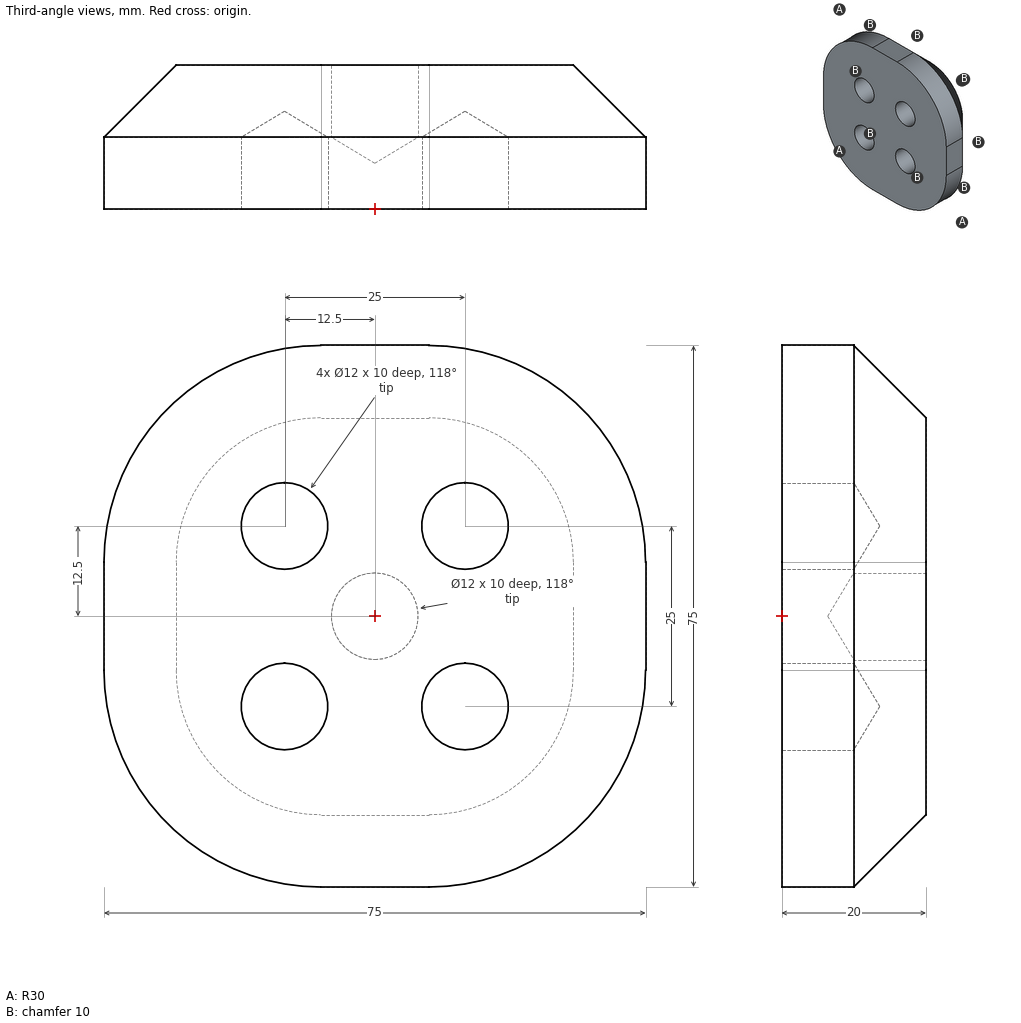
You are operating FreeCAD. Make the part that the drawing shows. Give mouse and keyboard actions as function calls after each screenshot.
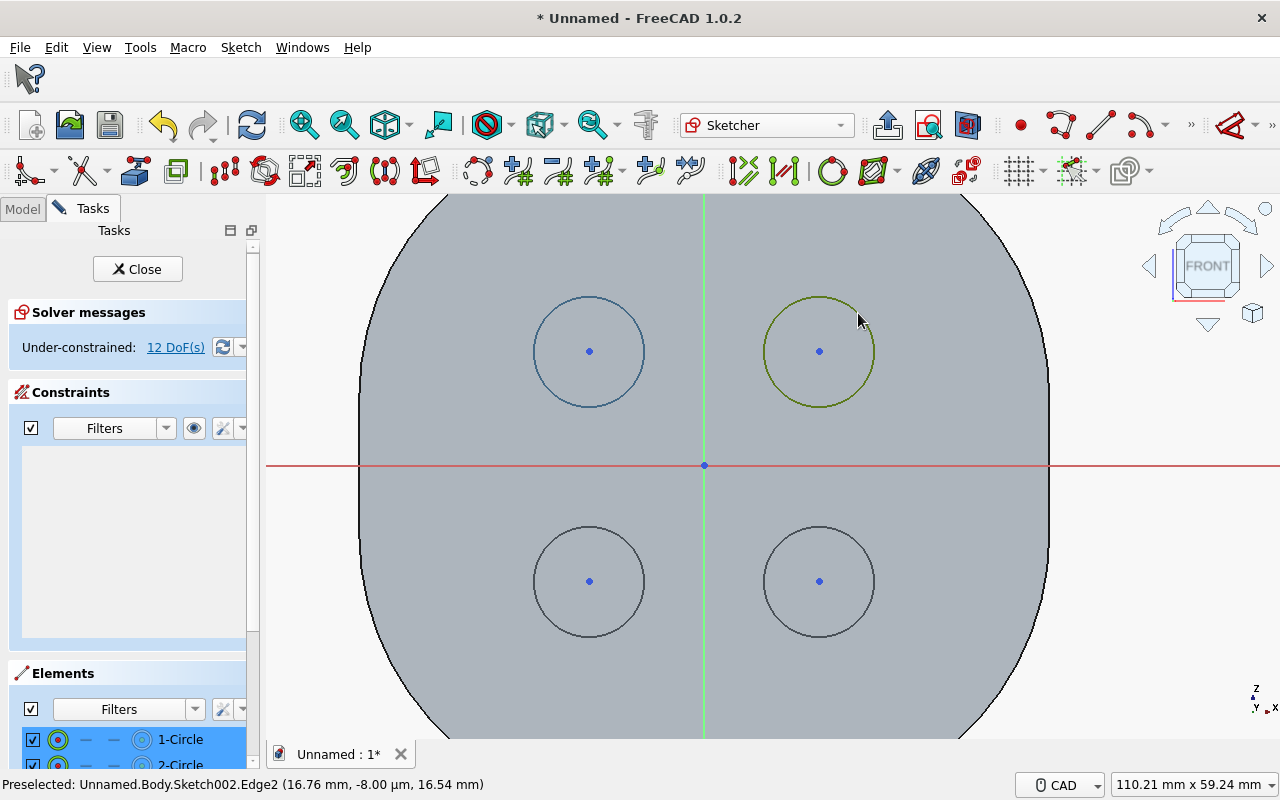
click(858, 543)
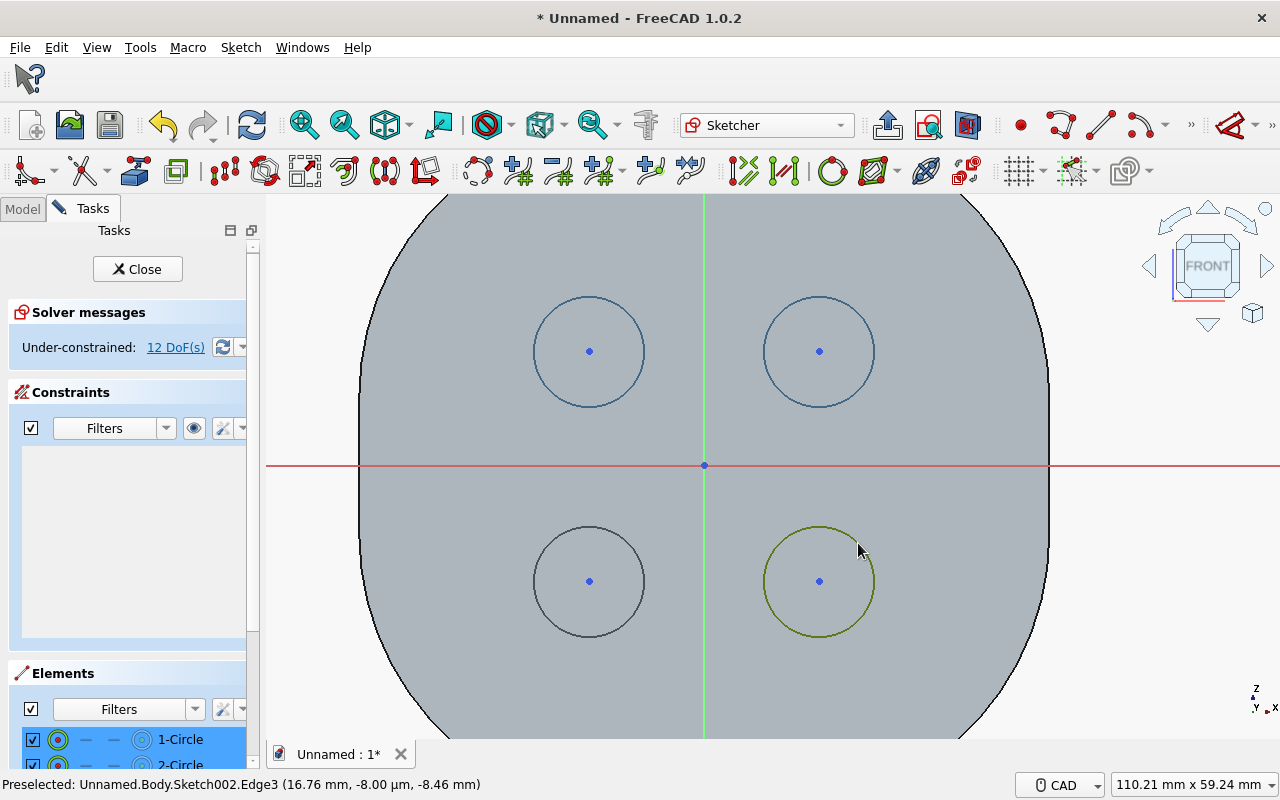
click(628, 543)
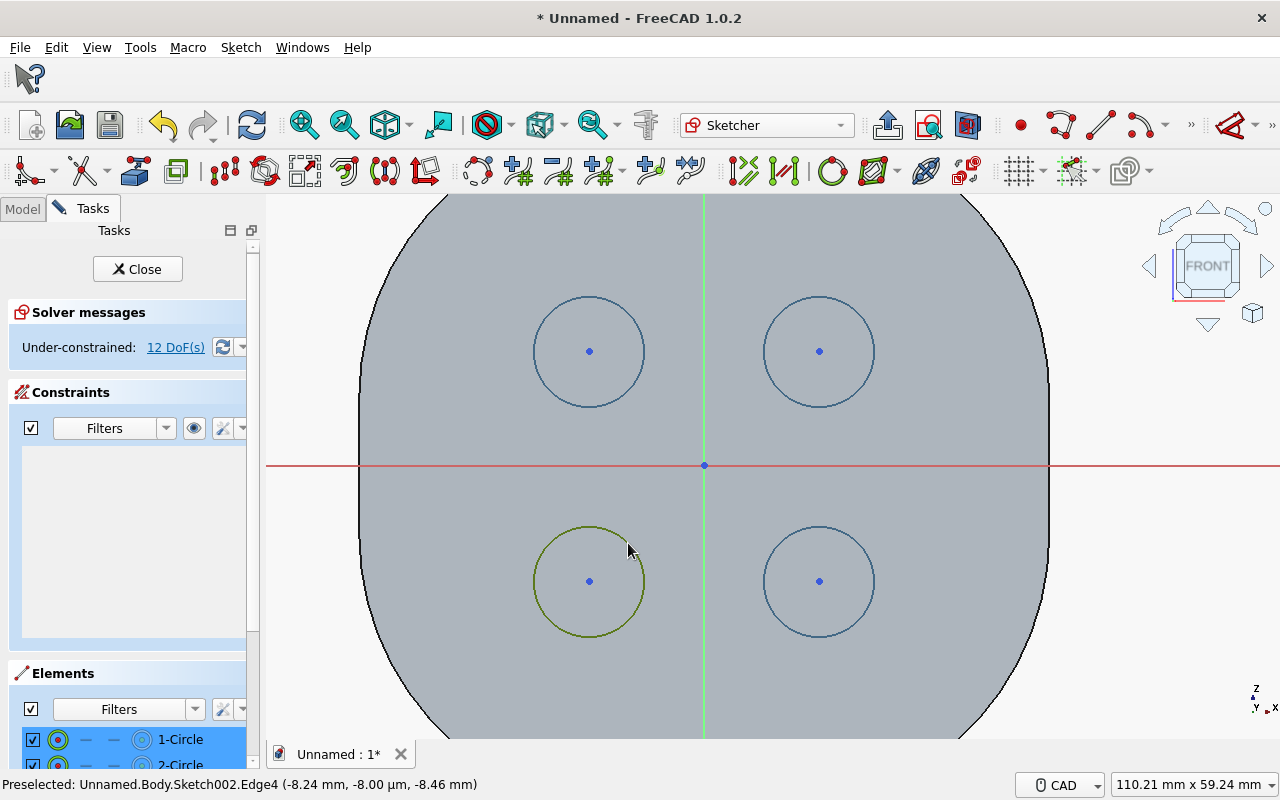
key(e)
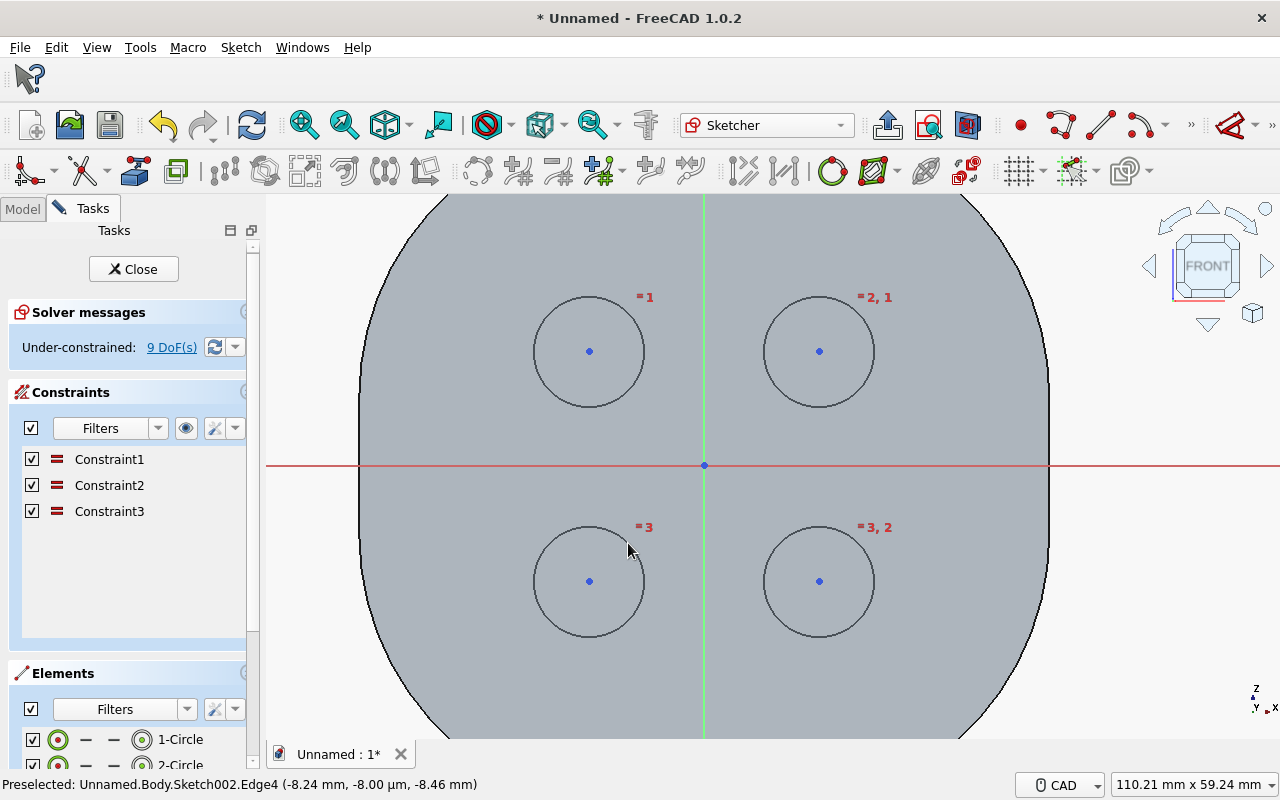
click(1230, 126)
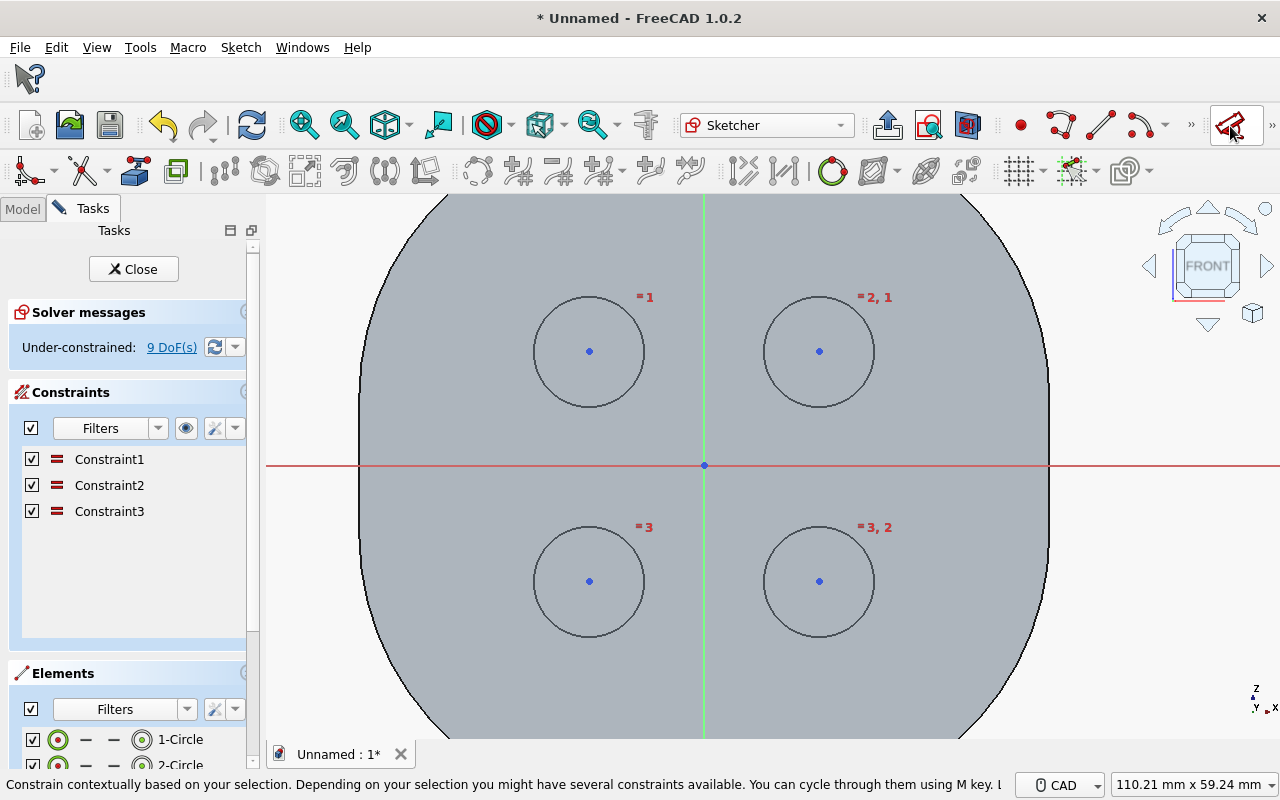
click(628, 313)
click(651, 290)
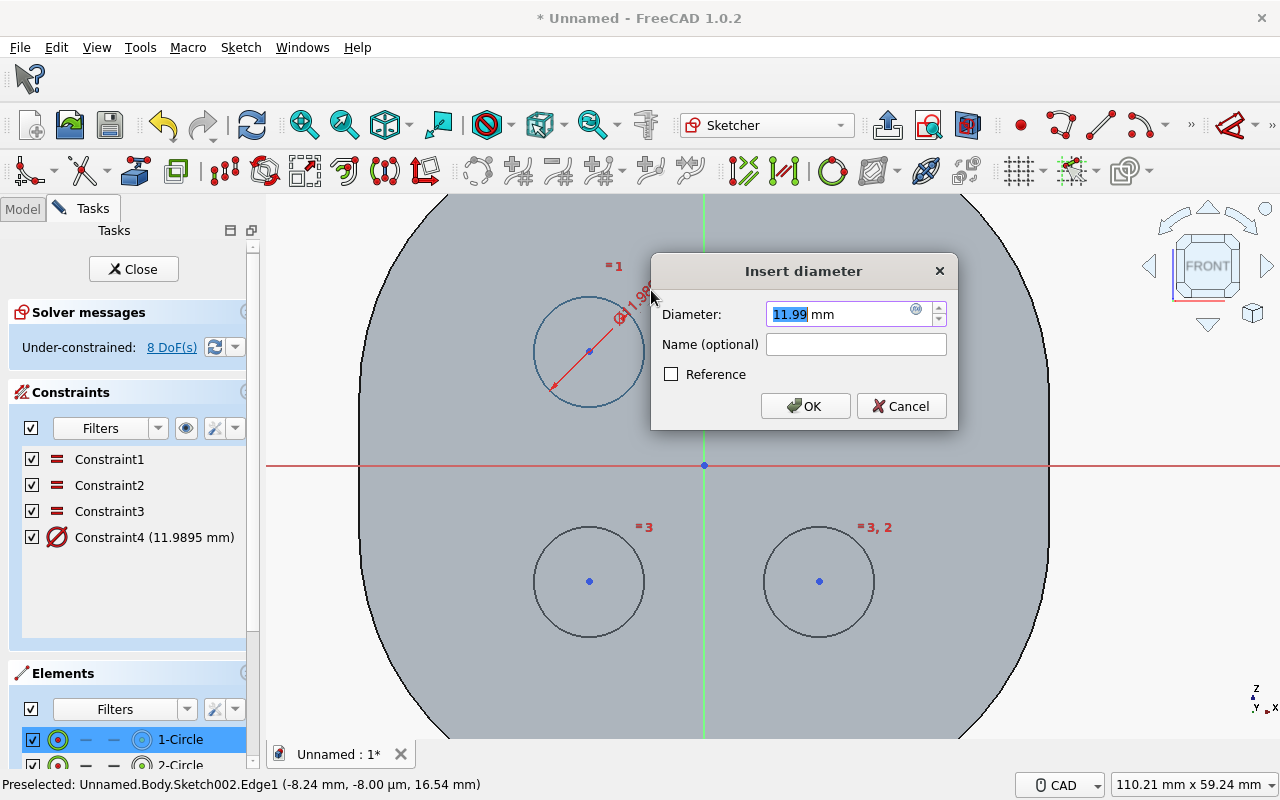
text(12)
key(Return)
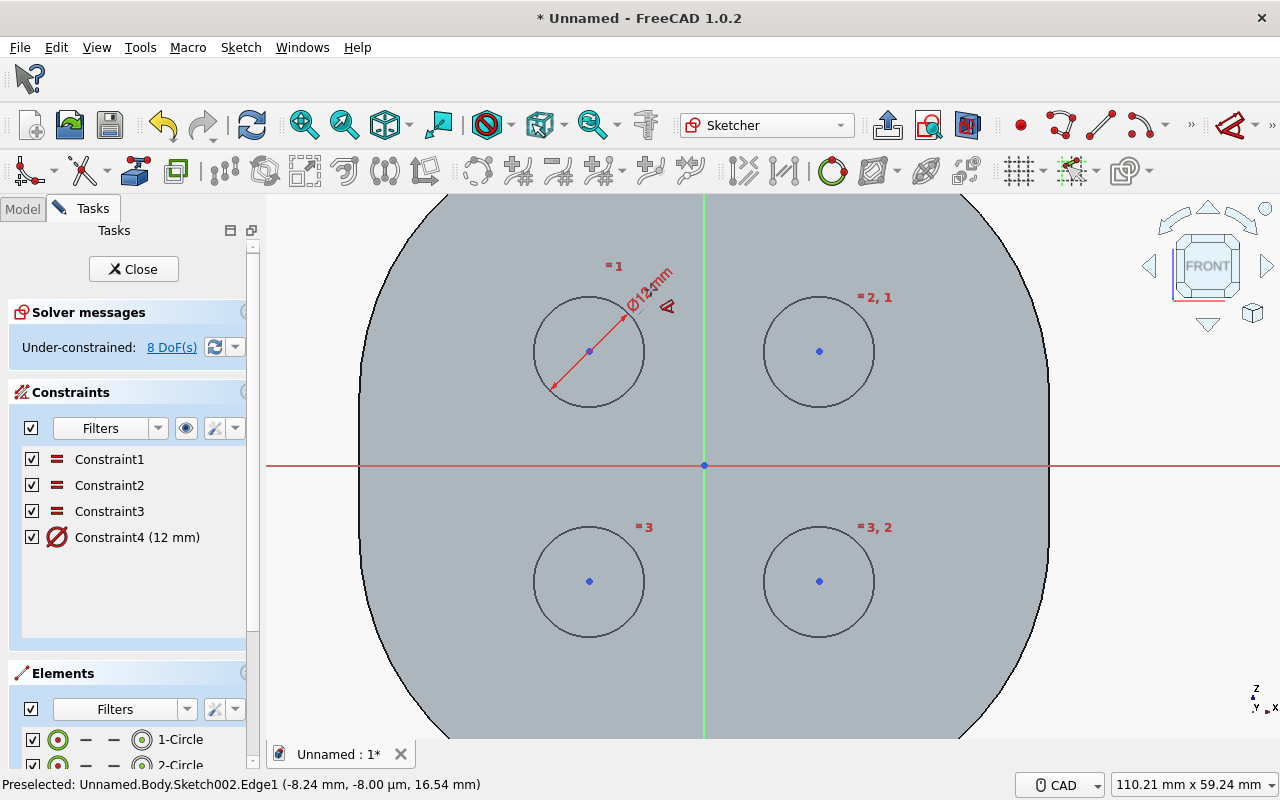
click(589, 352)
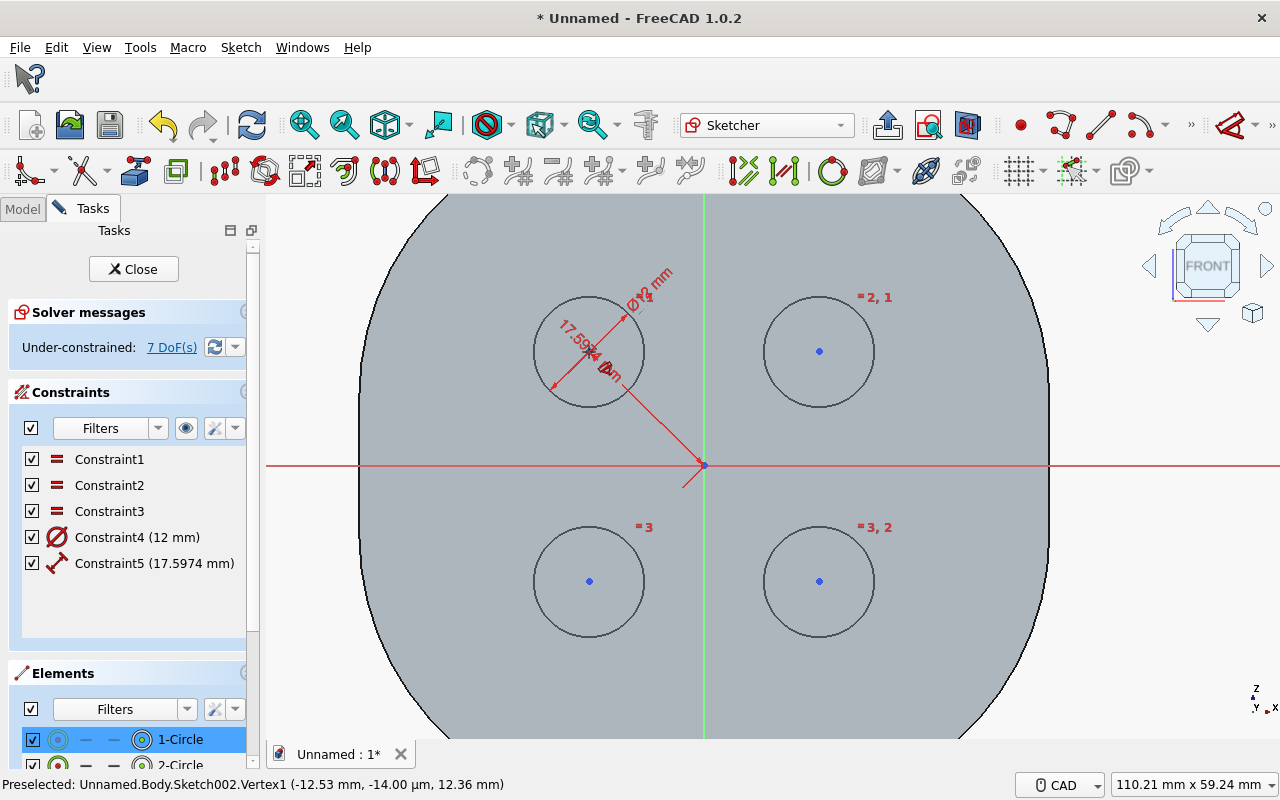
click(819, 352)
click(651, 318)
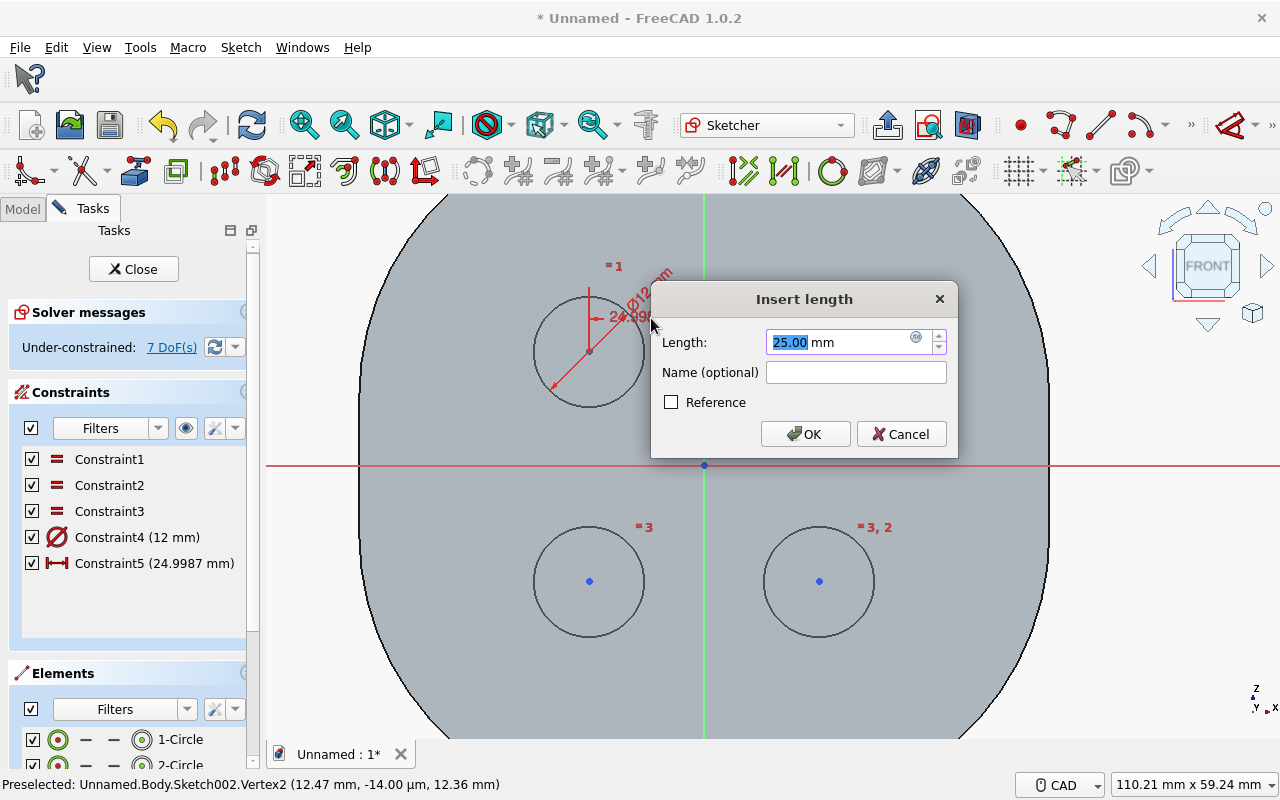
text(25)
key(Return)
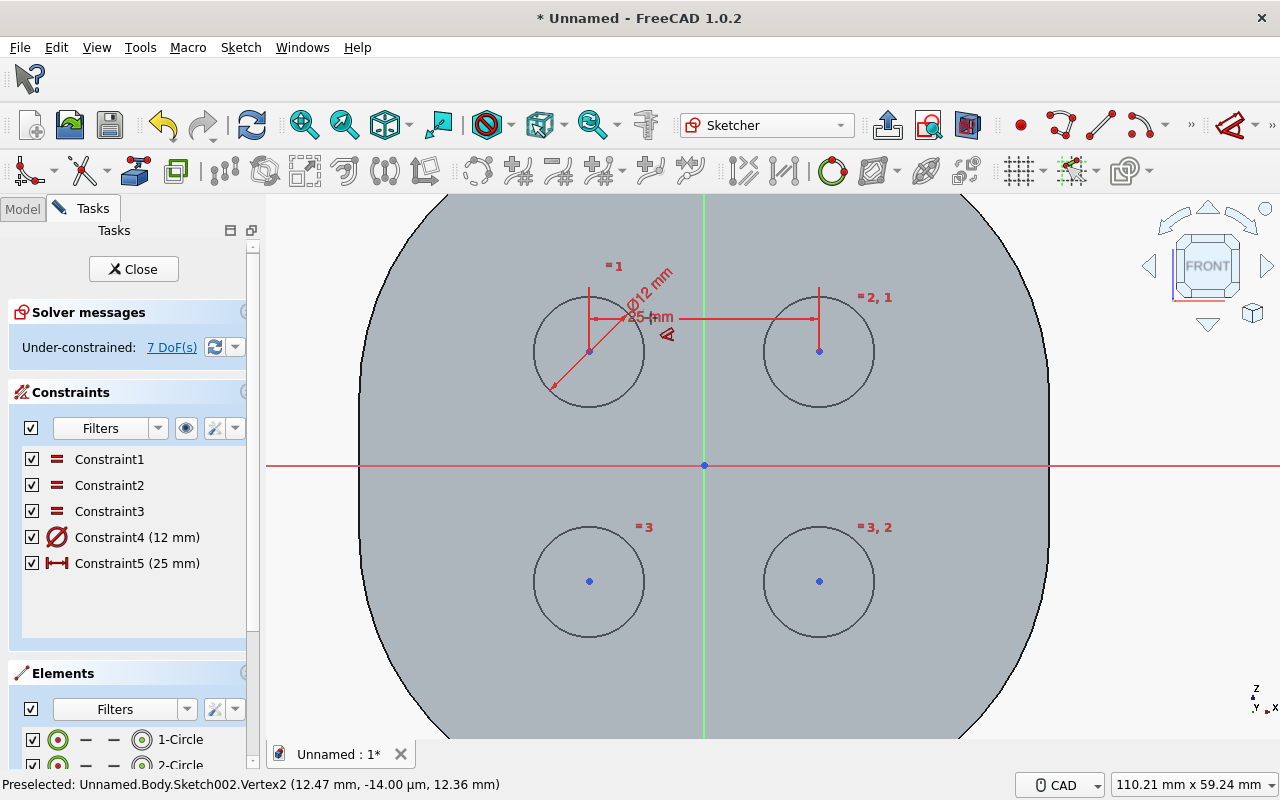
click(589, 352)